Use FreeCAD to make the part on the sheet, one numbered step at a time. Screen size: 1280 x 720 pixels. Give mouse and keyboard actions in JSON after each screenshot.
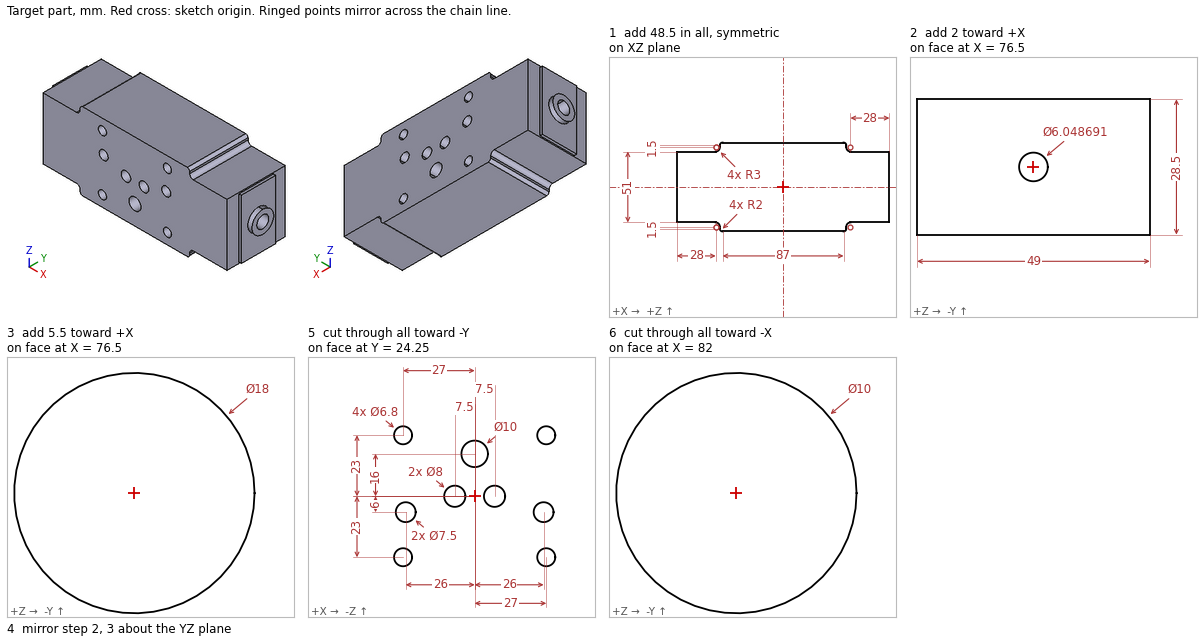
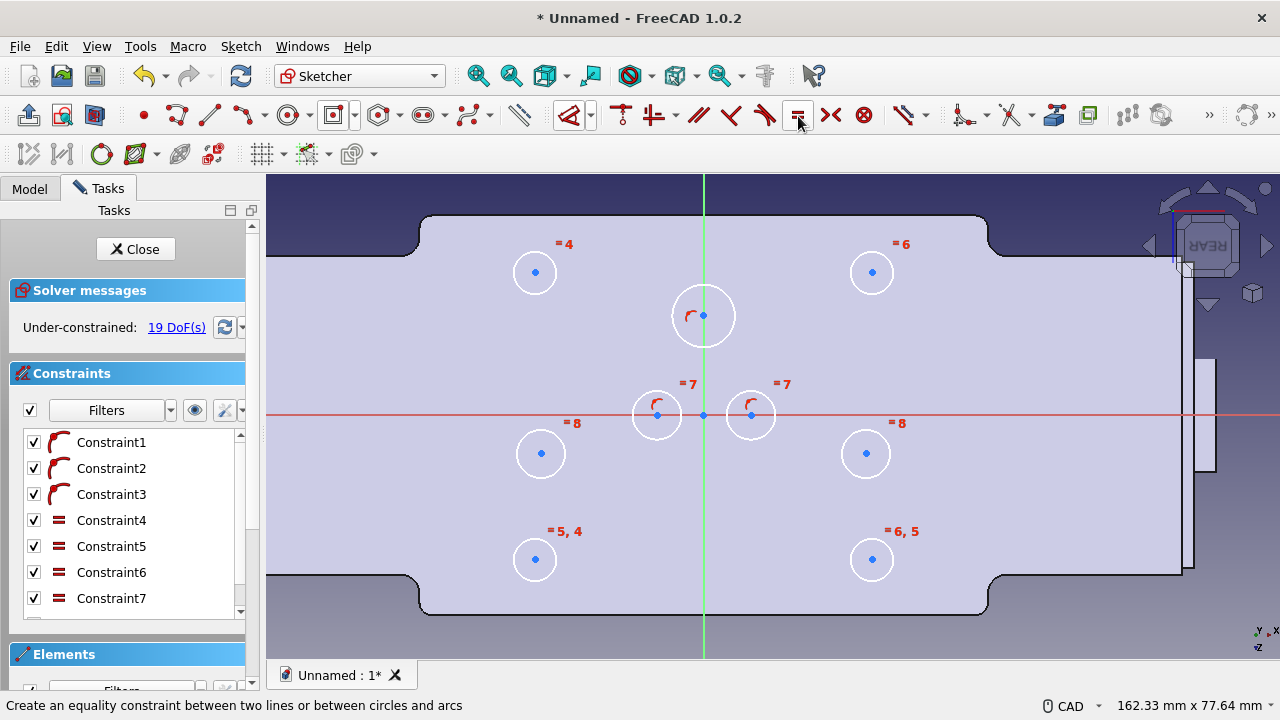
{"action": "left_click", "coordinate": [535, 273]}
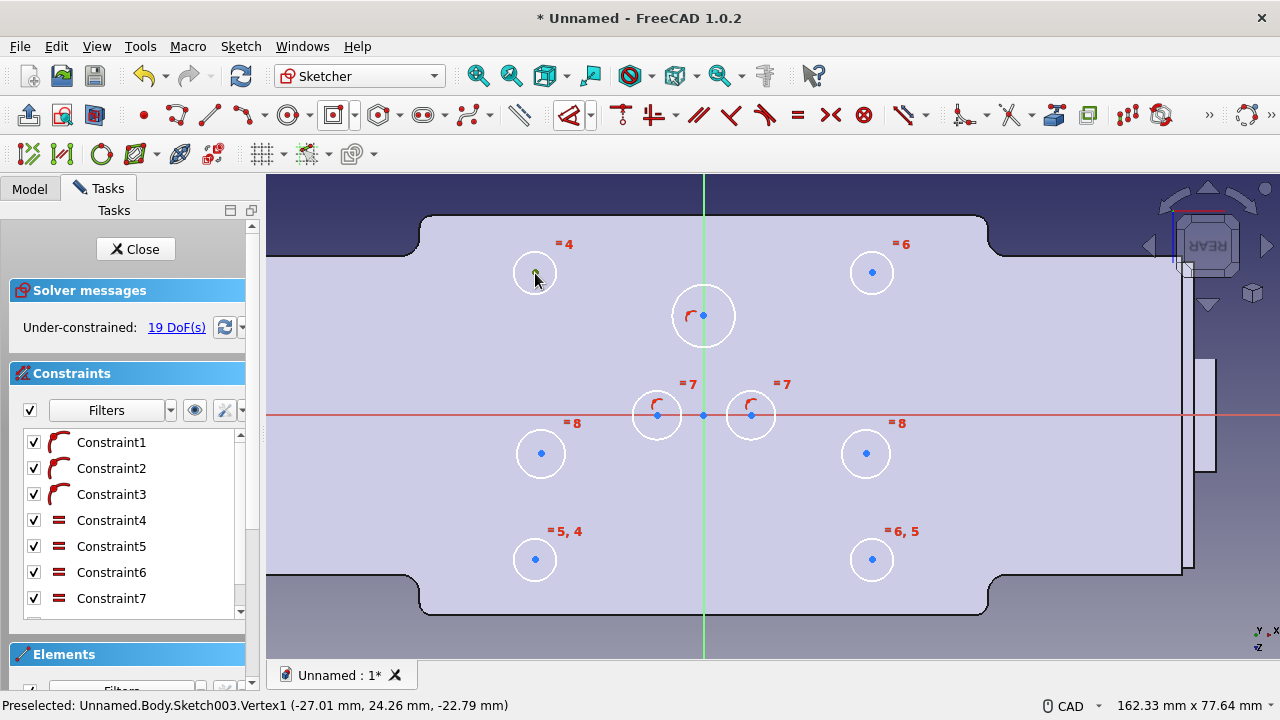
{"action": "left_click", "coordinate": [535, 560]}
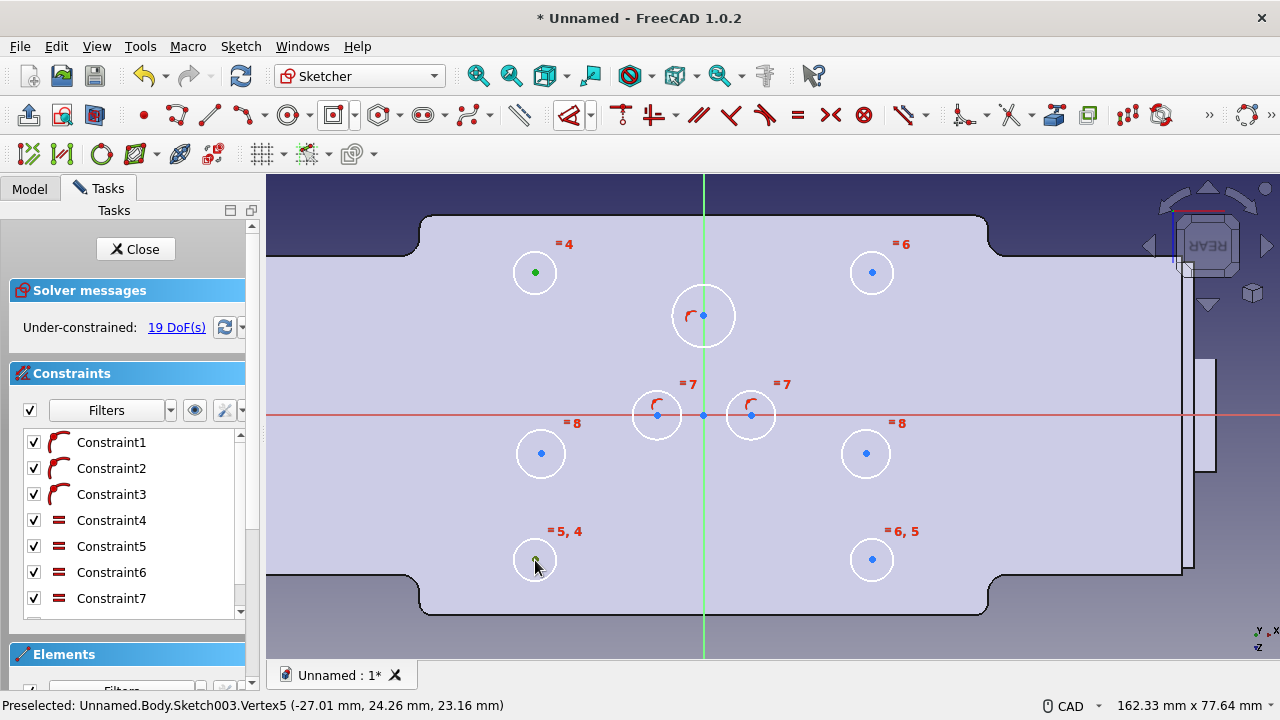
{"action": "key", "text": "v"}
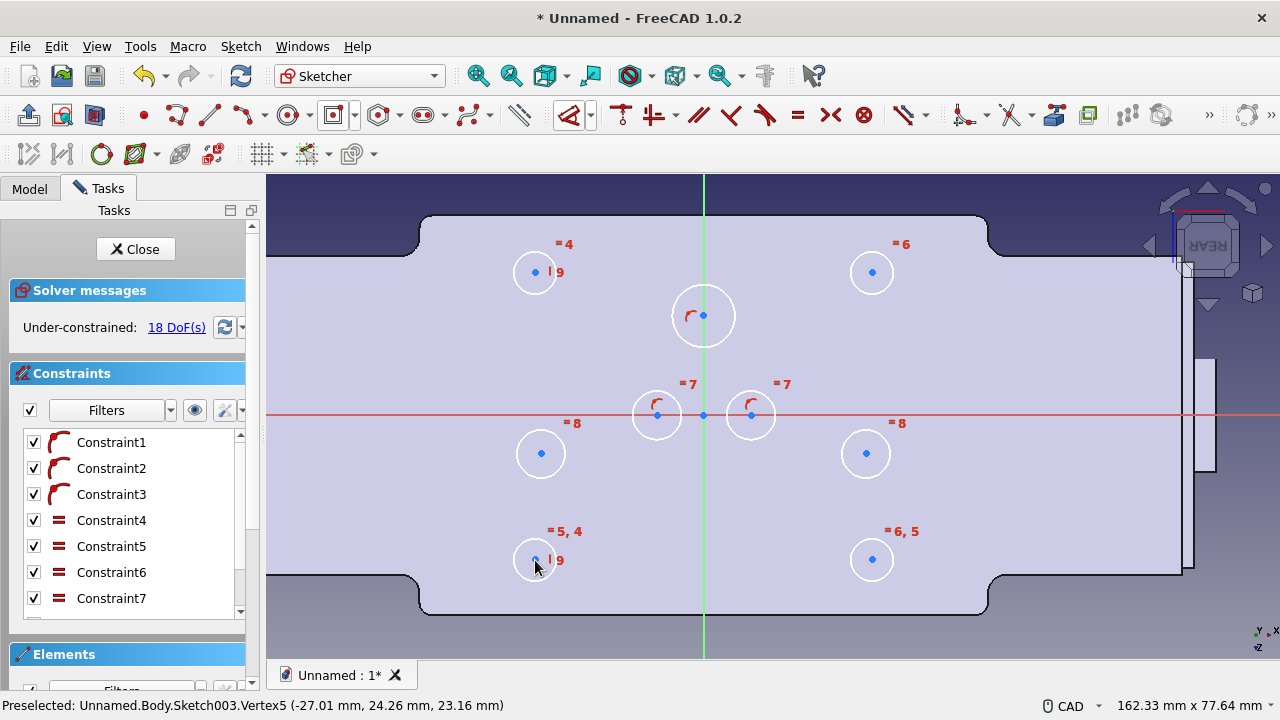
{"action": "left_click", "coordinate": [535, 560]}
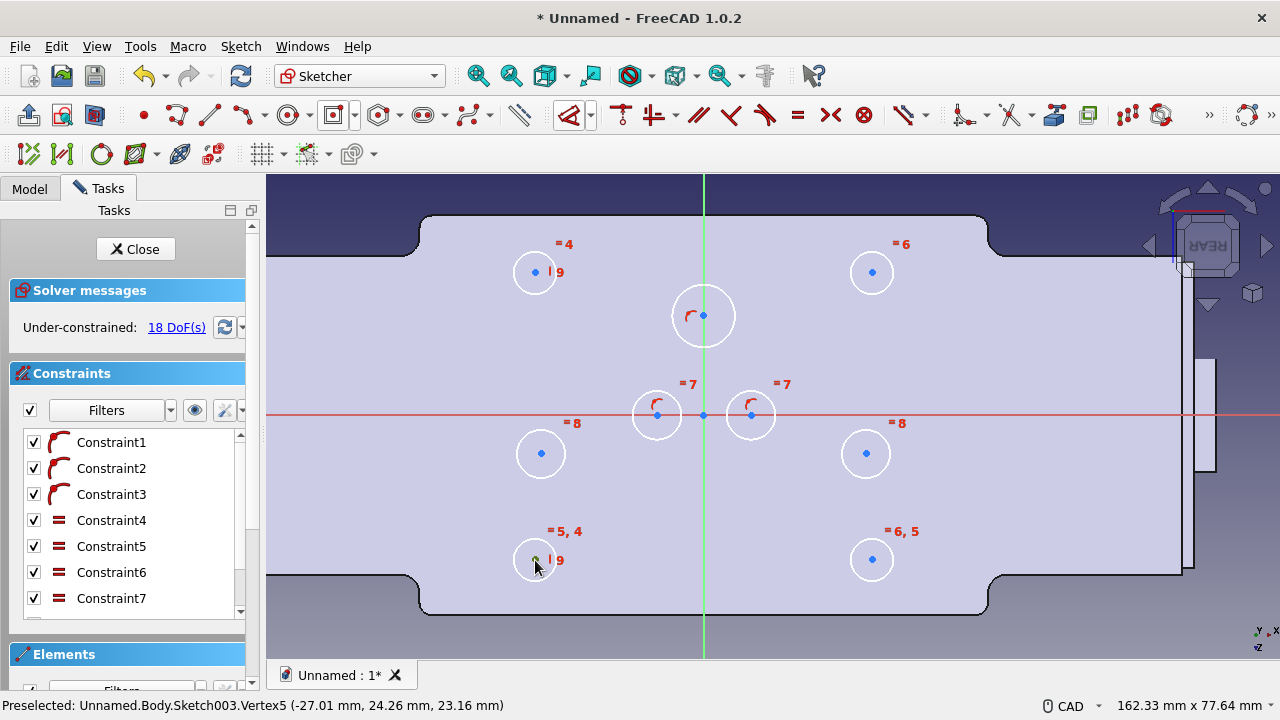
{"action": "left_click", "coordinate": [872, 560]}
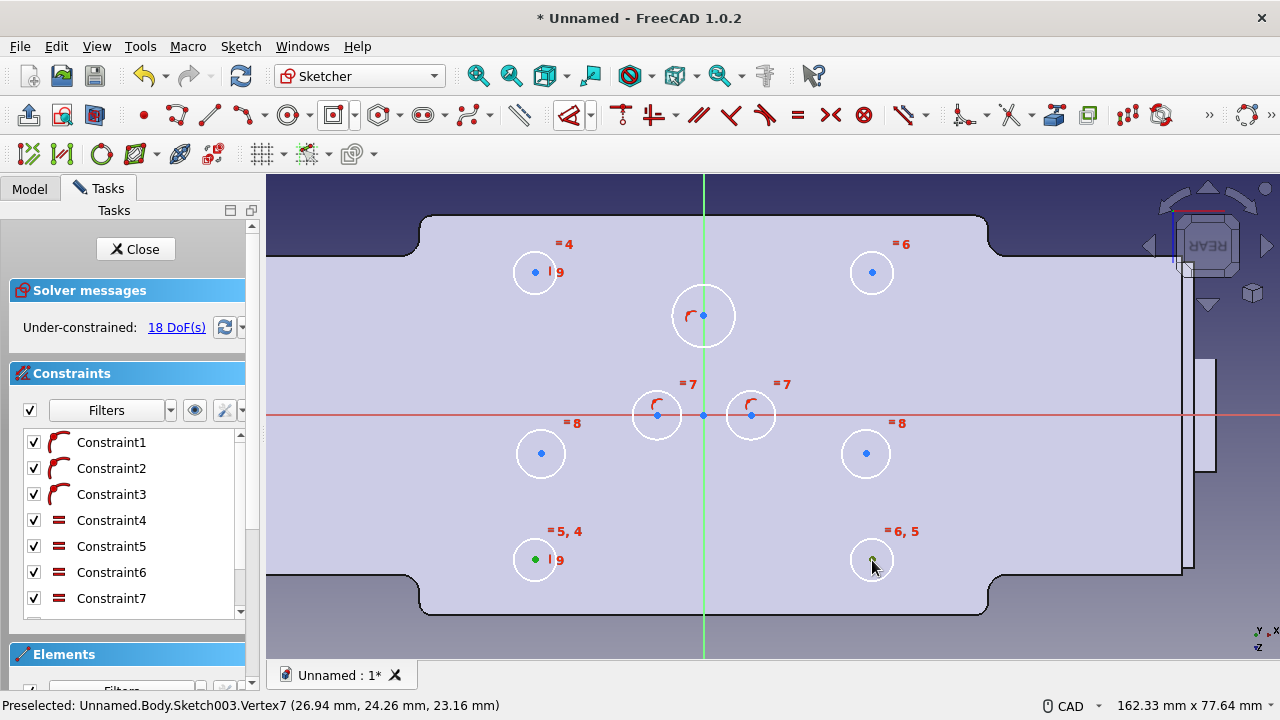
{"action": "left_click", "coordinate": [676, 116]}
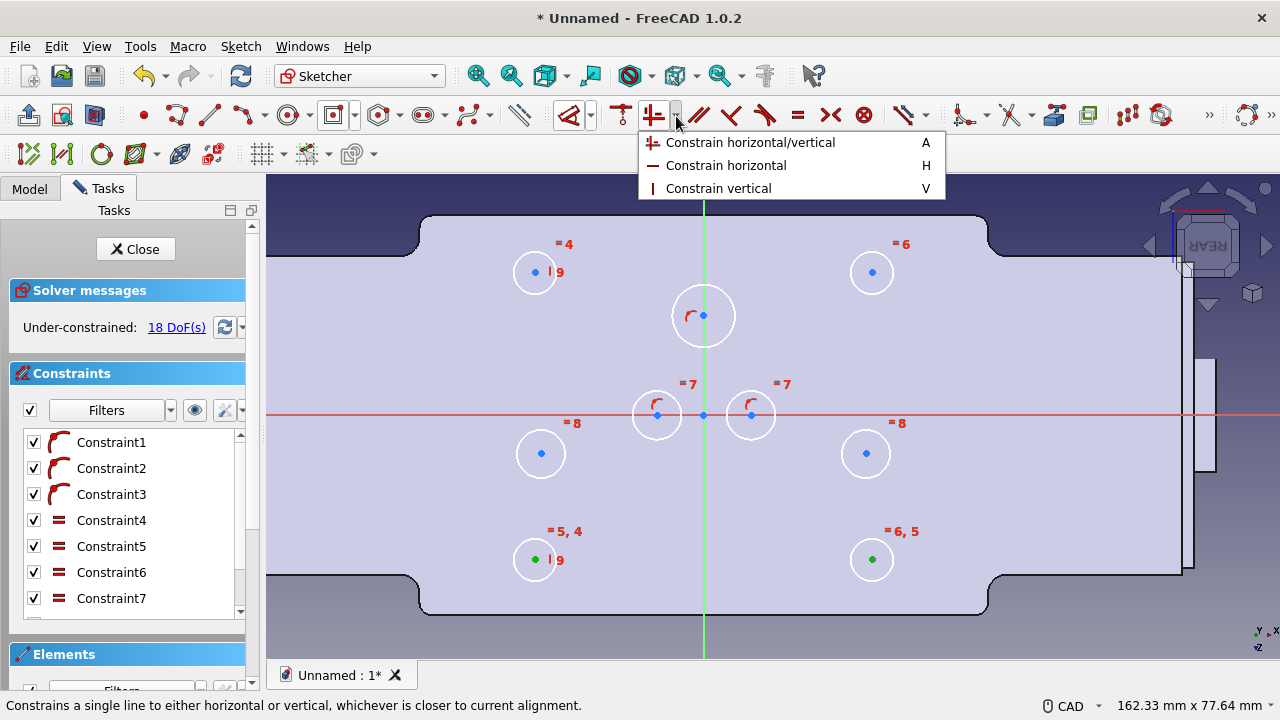
{"action": "left_click", "coordinate": [792, 166]}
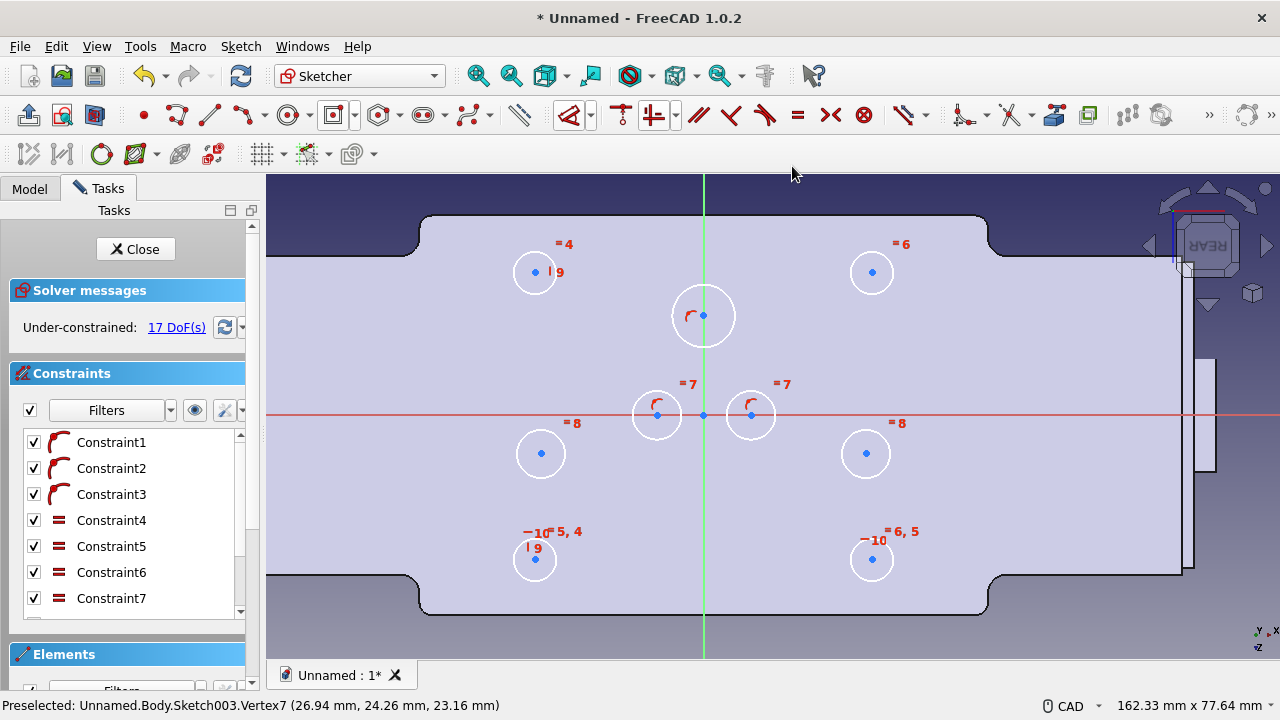
{"action": "left_click", "coordinate": [541, 454]}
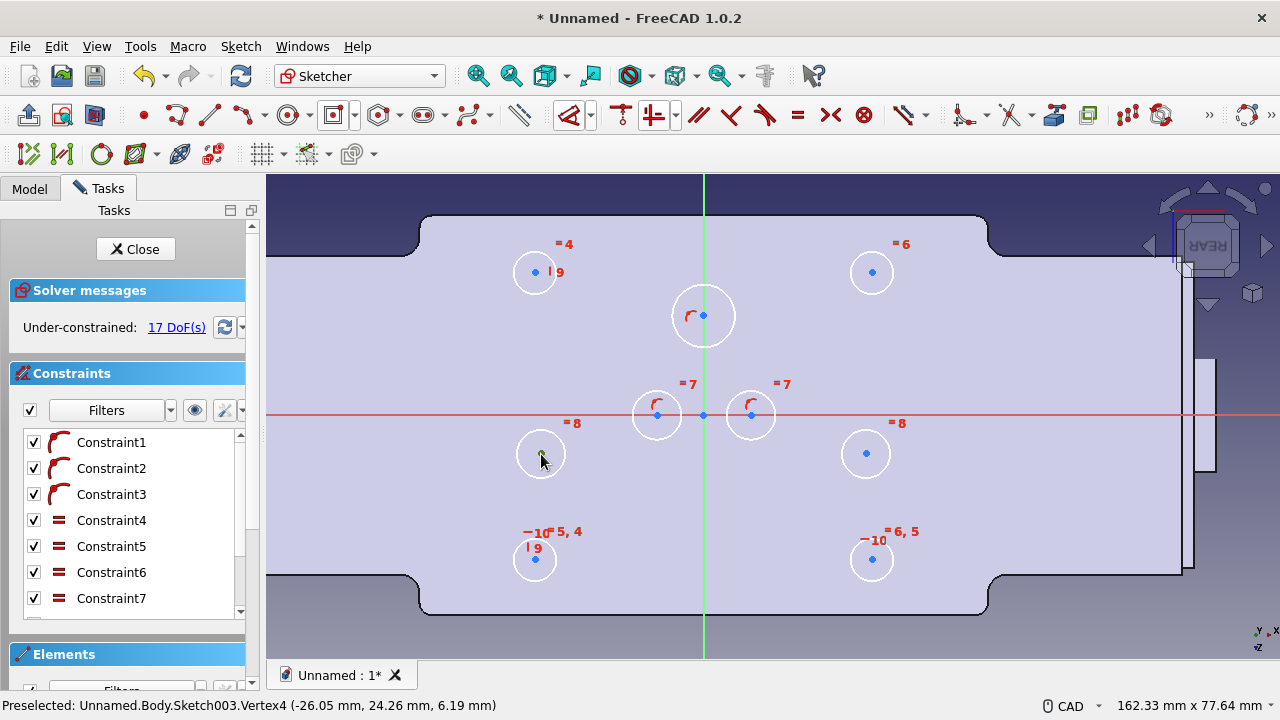
{"action": "left_click", "coordinate": [866, 454]}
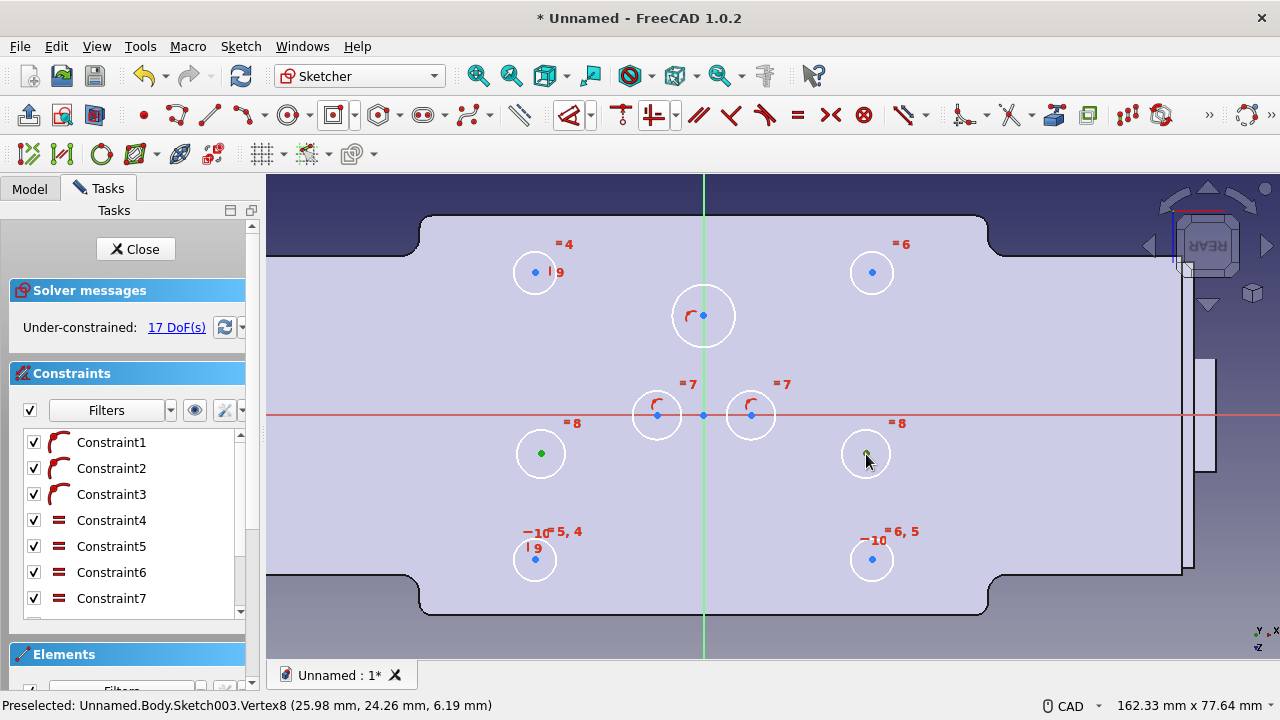
{"action": "left_click", "coordinate": [676, 116]}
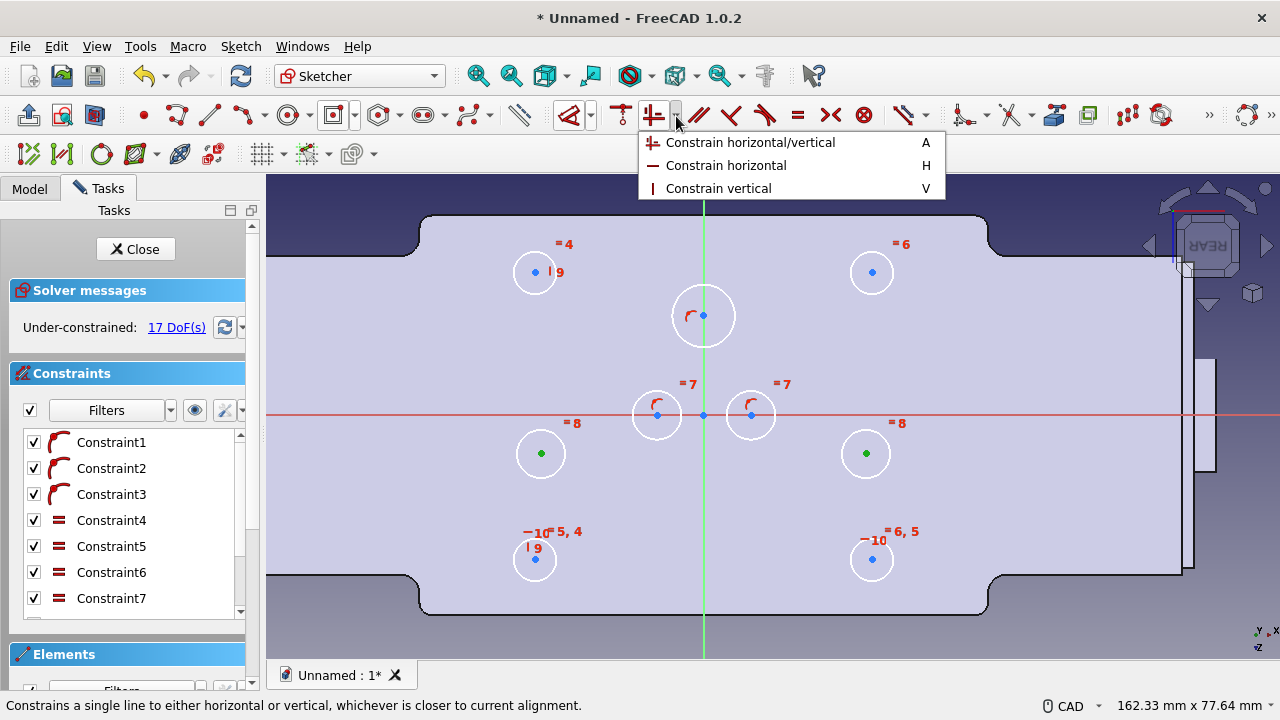
{"action": "left_click", "coordinate": [792, 166]}